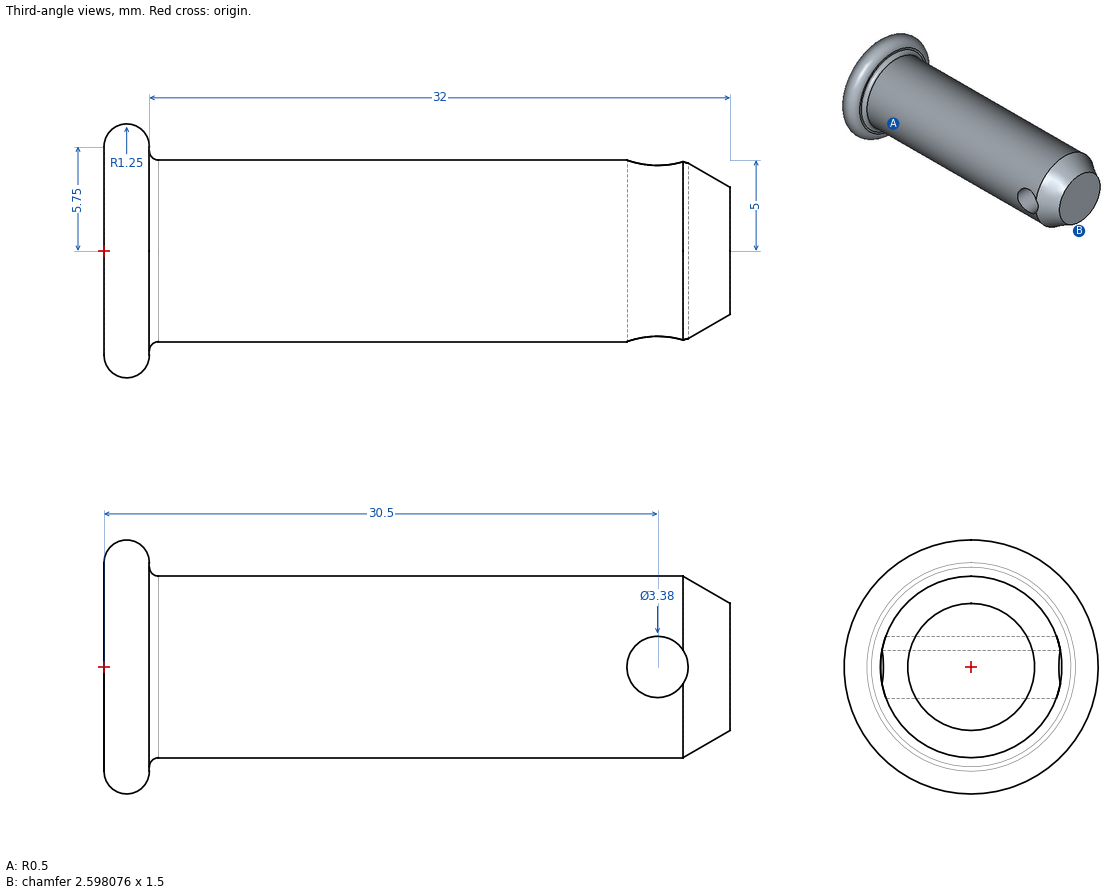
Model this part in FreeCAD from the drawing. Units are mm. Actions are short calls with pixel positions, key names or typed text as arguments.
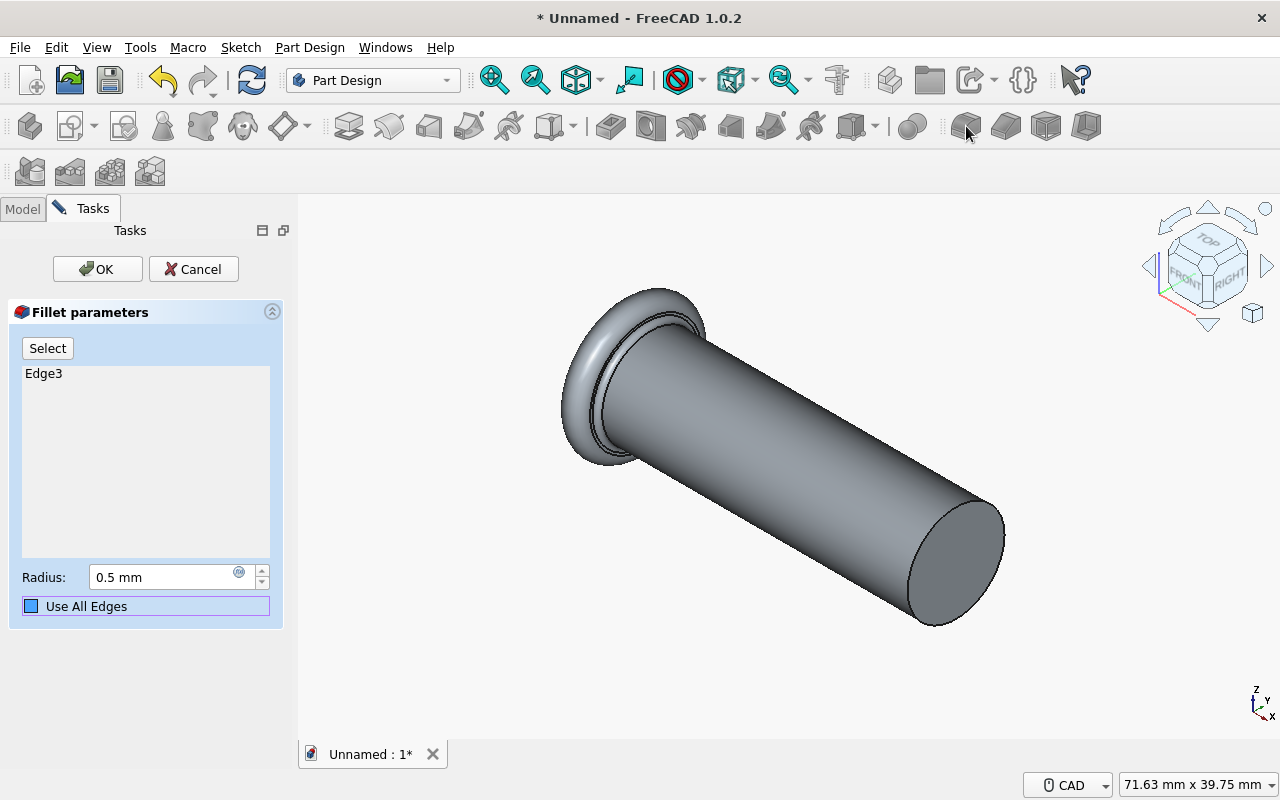
click(98, 269)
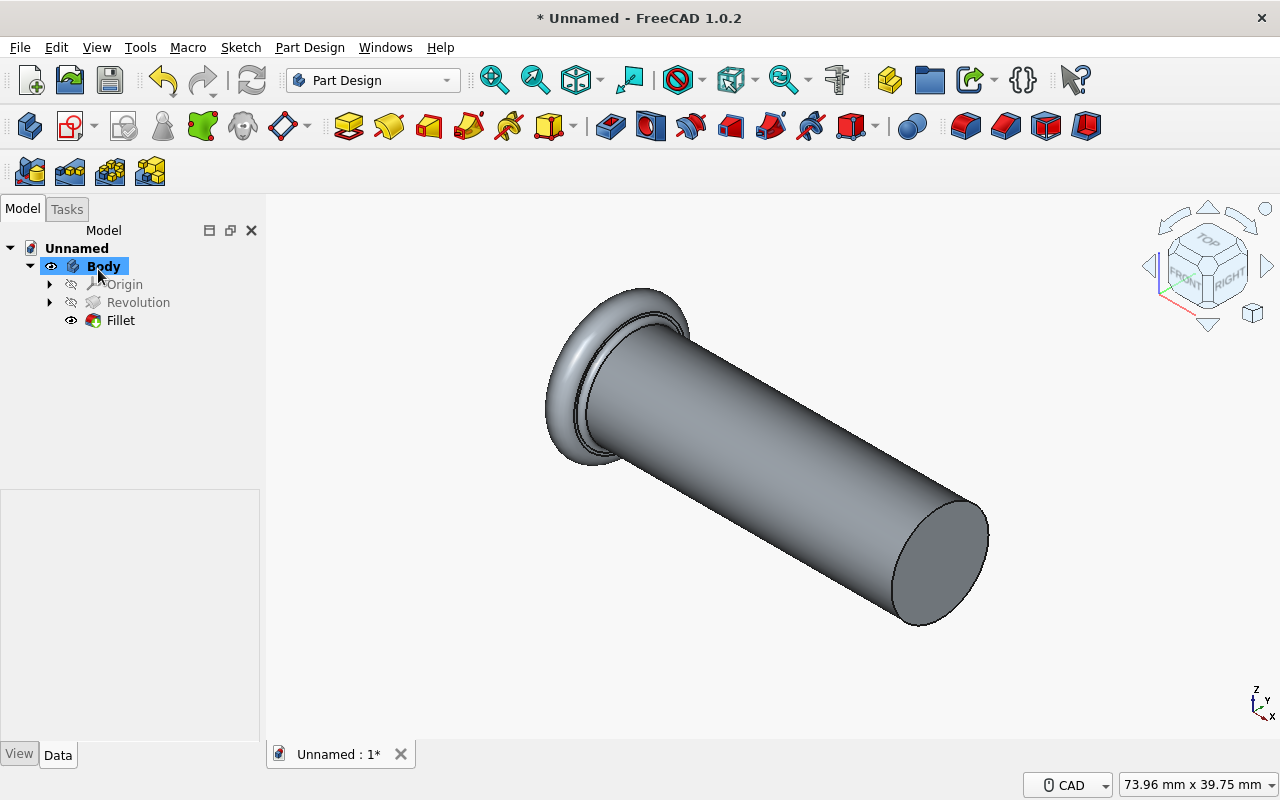
click(892, 590)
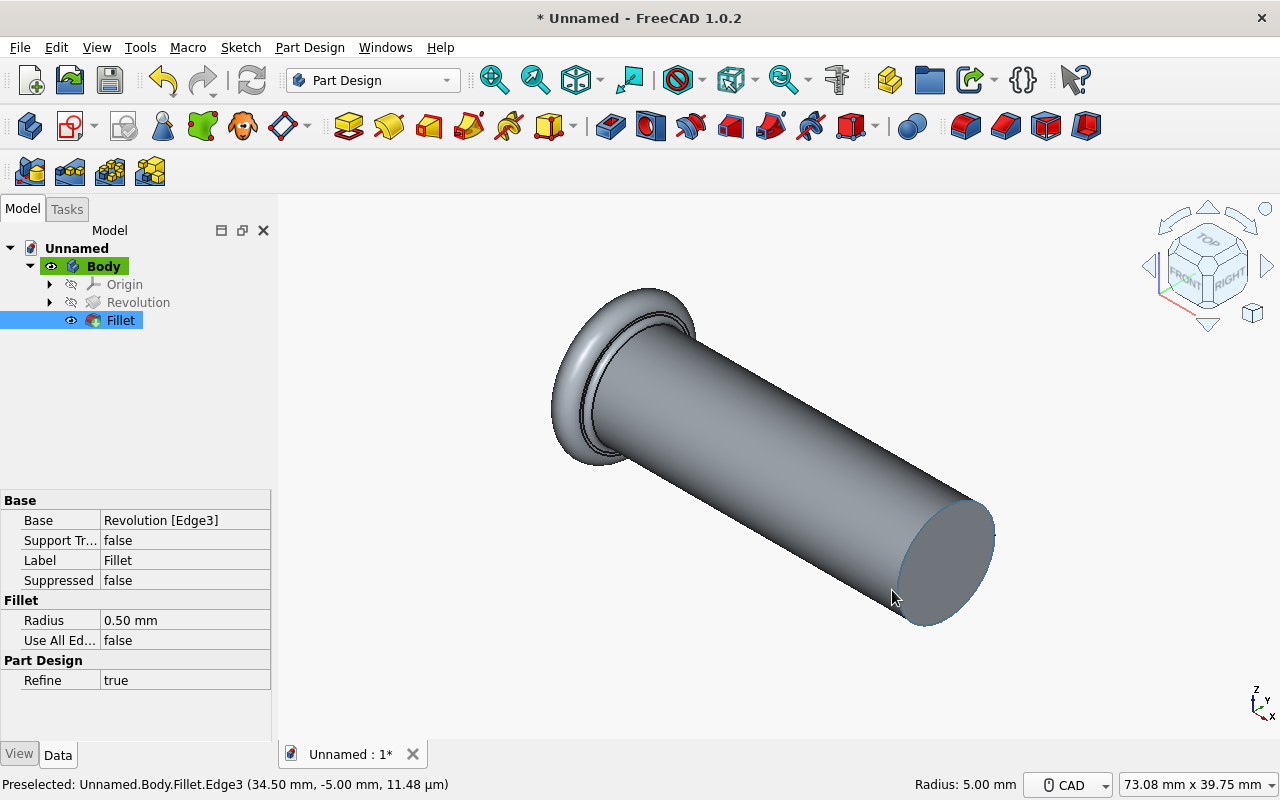
click(1006, 126)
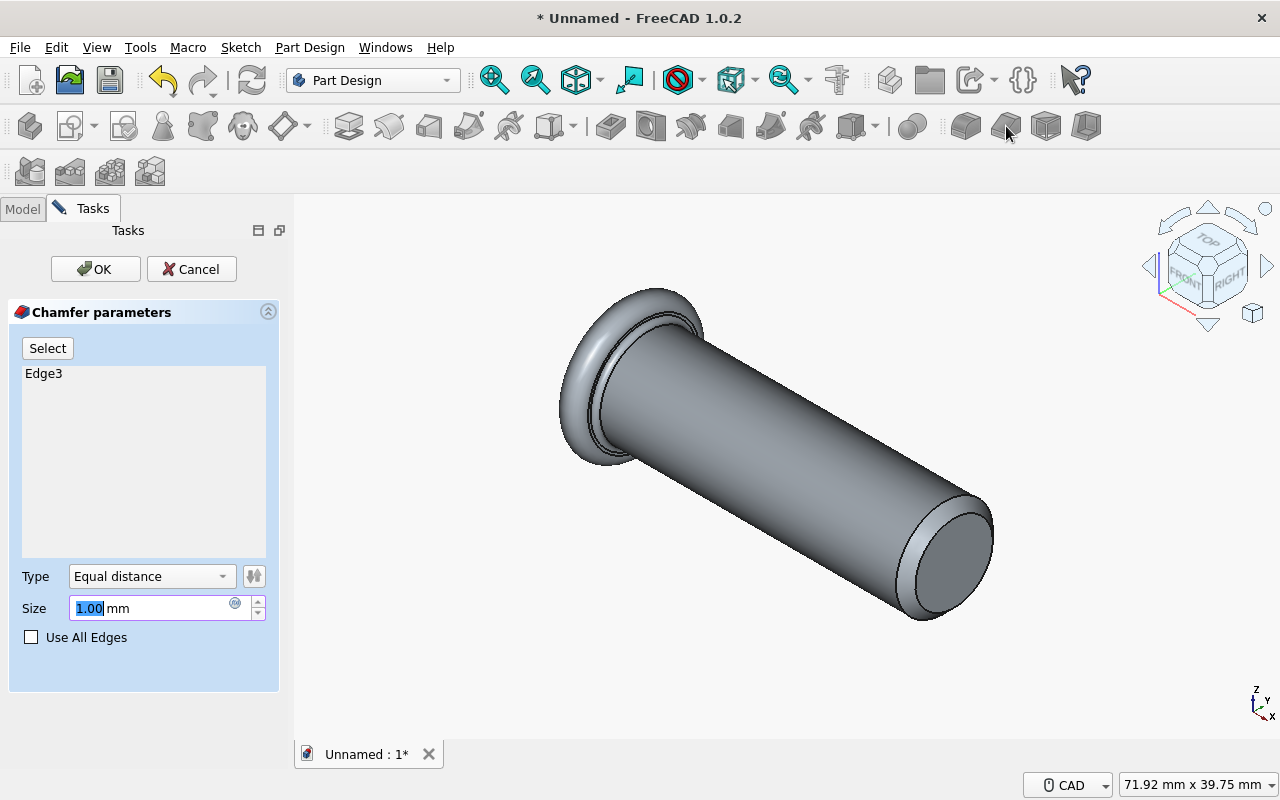
text(2.598076)
key(Tab)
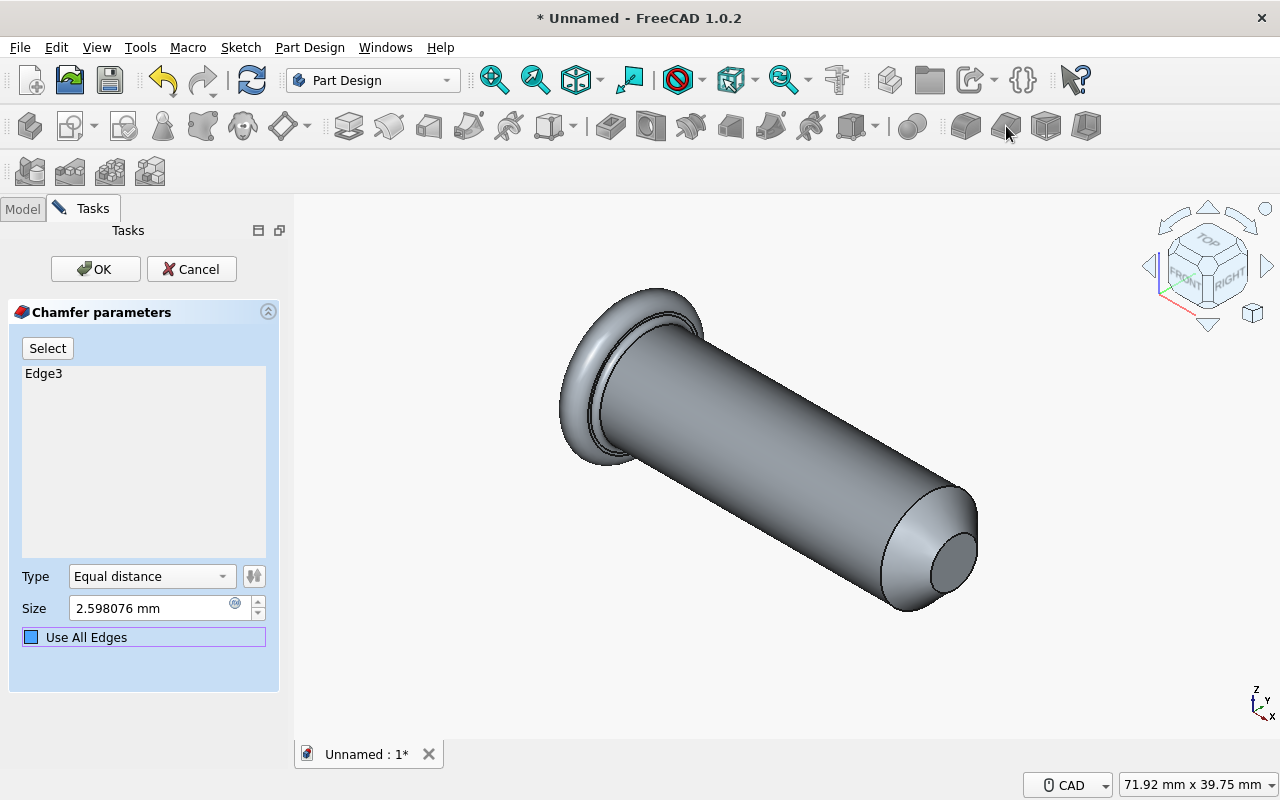
click(153, 576)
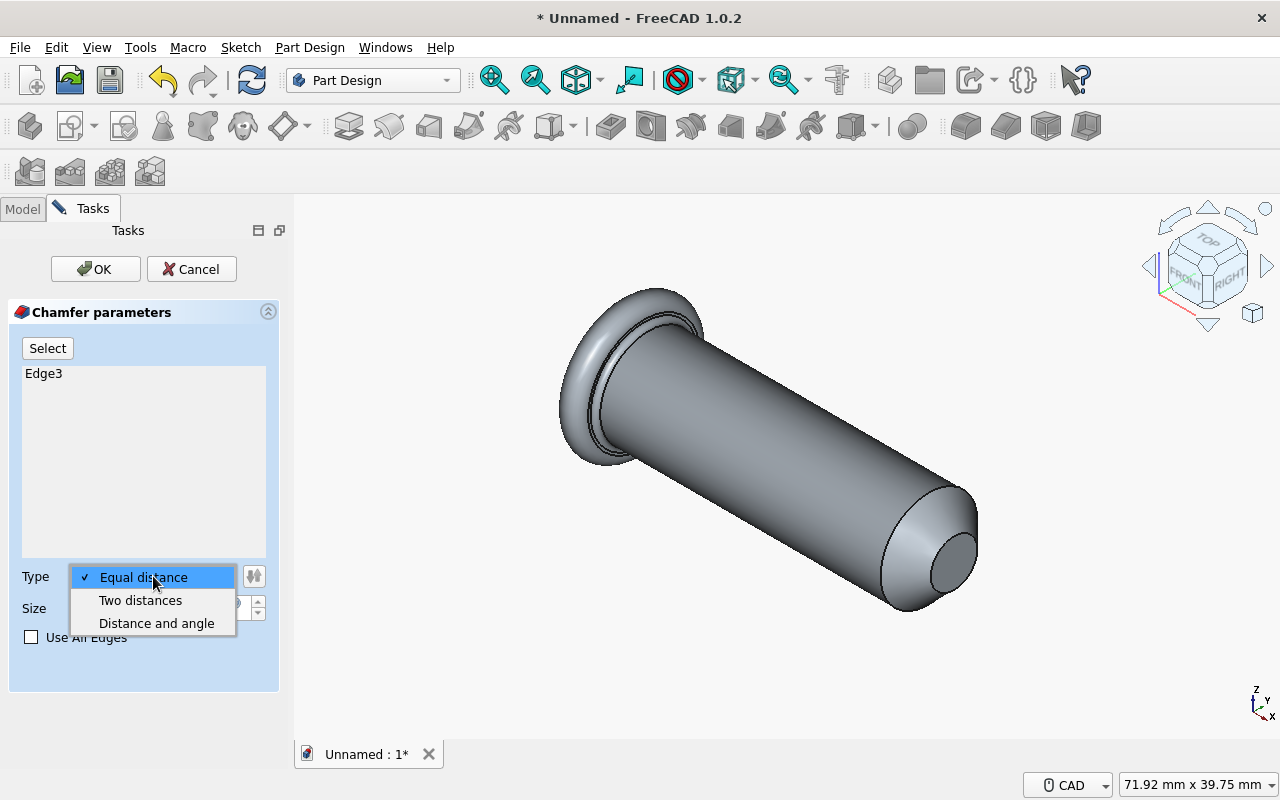
click(152, 600)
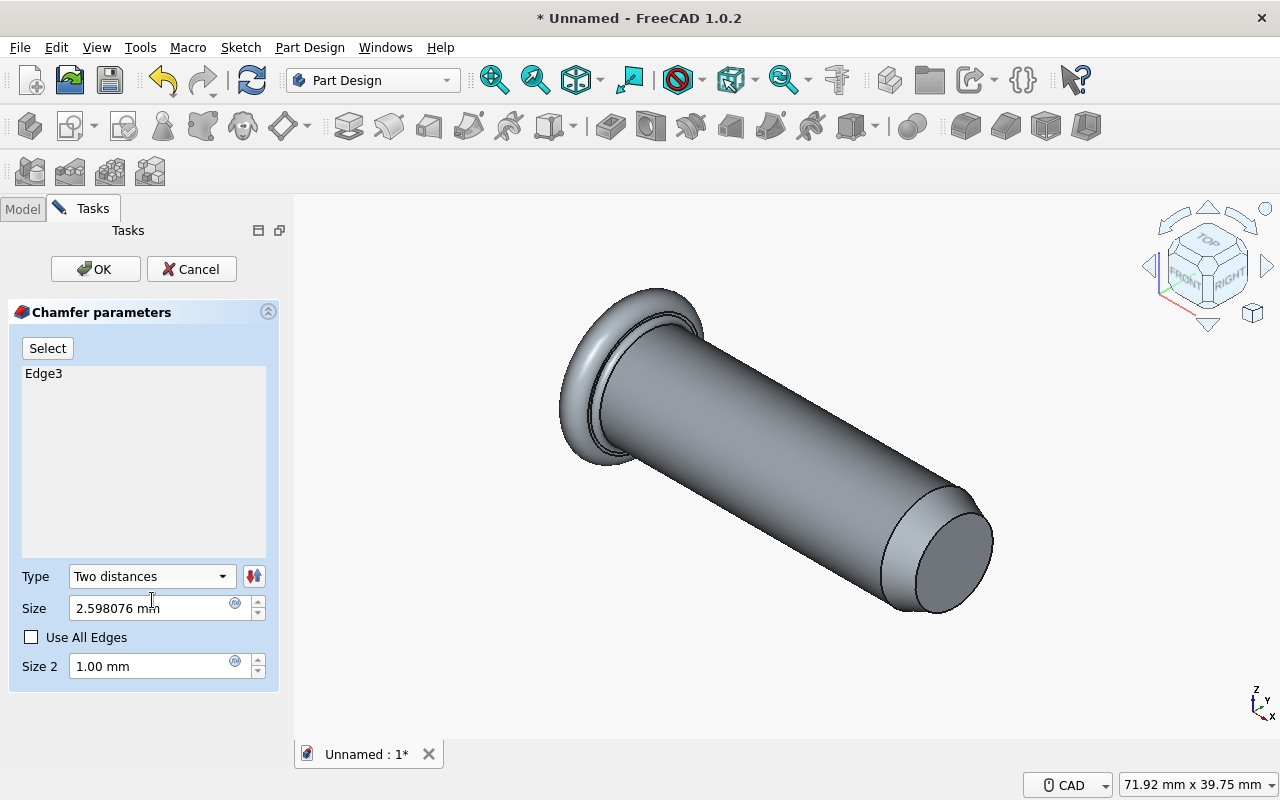
triple_click(160, 666)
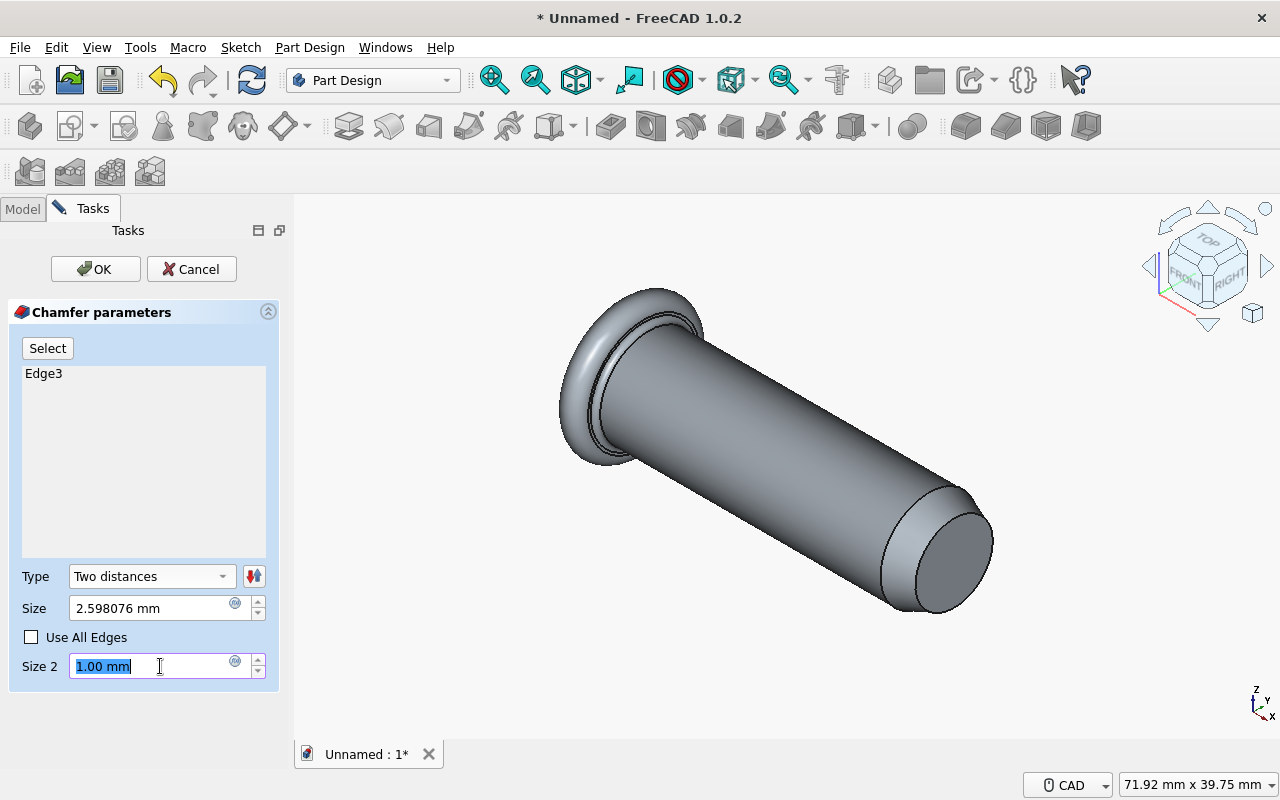
text(1.5)
key(Tab)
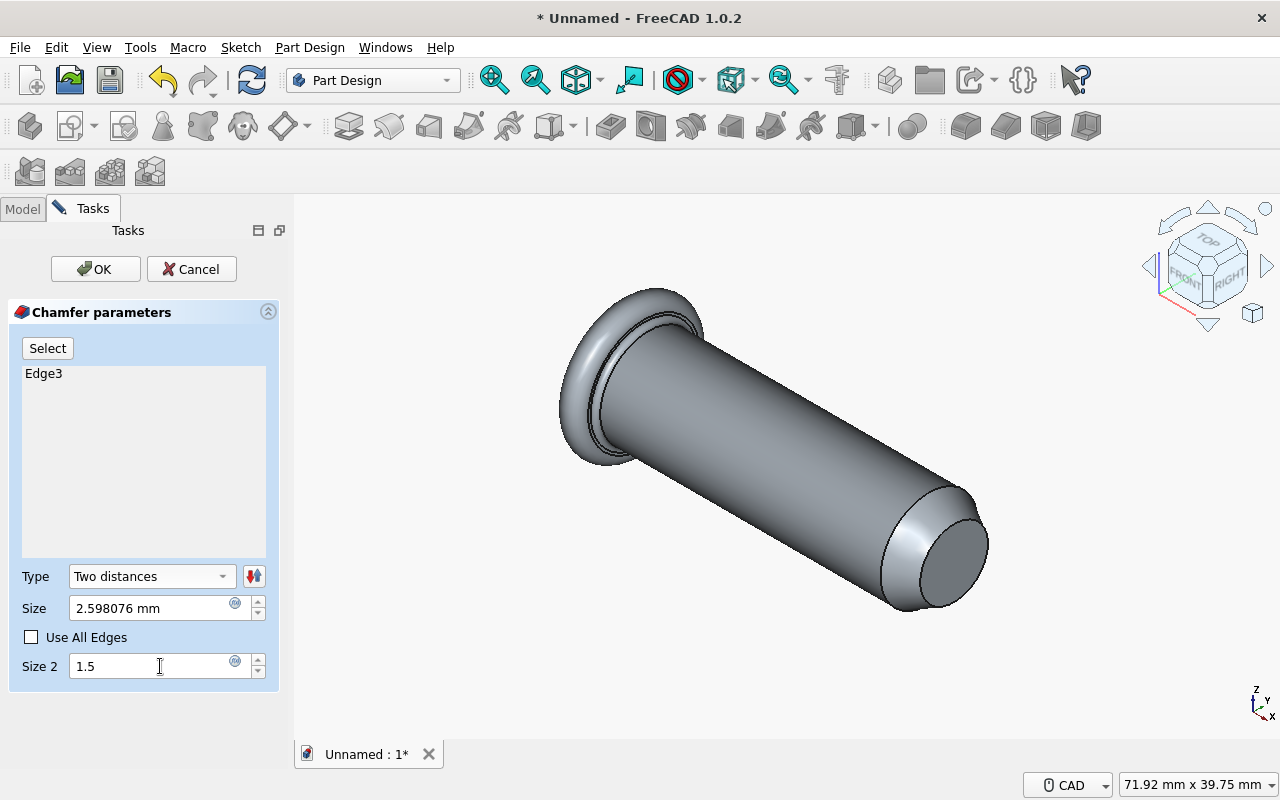
click(96, 269)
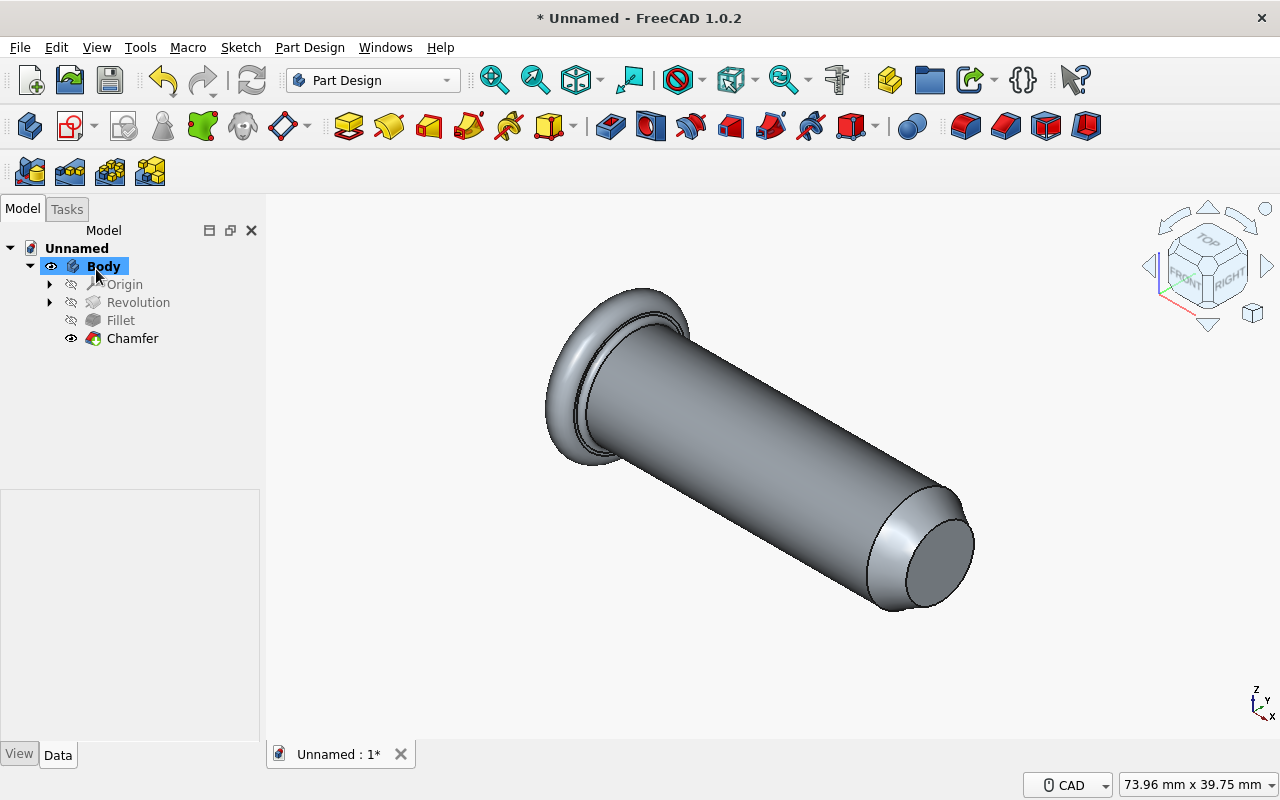
click(70, 126)